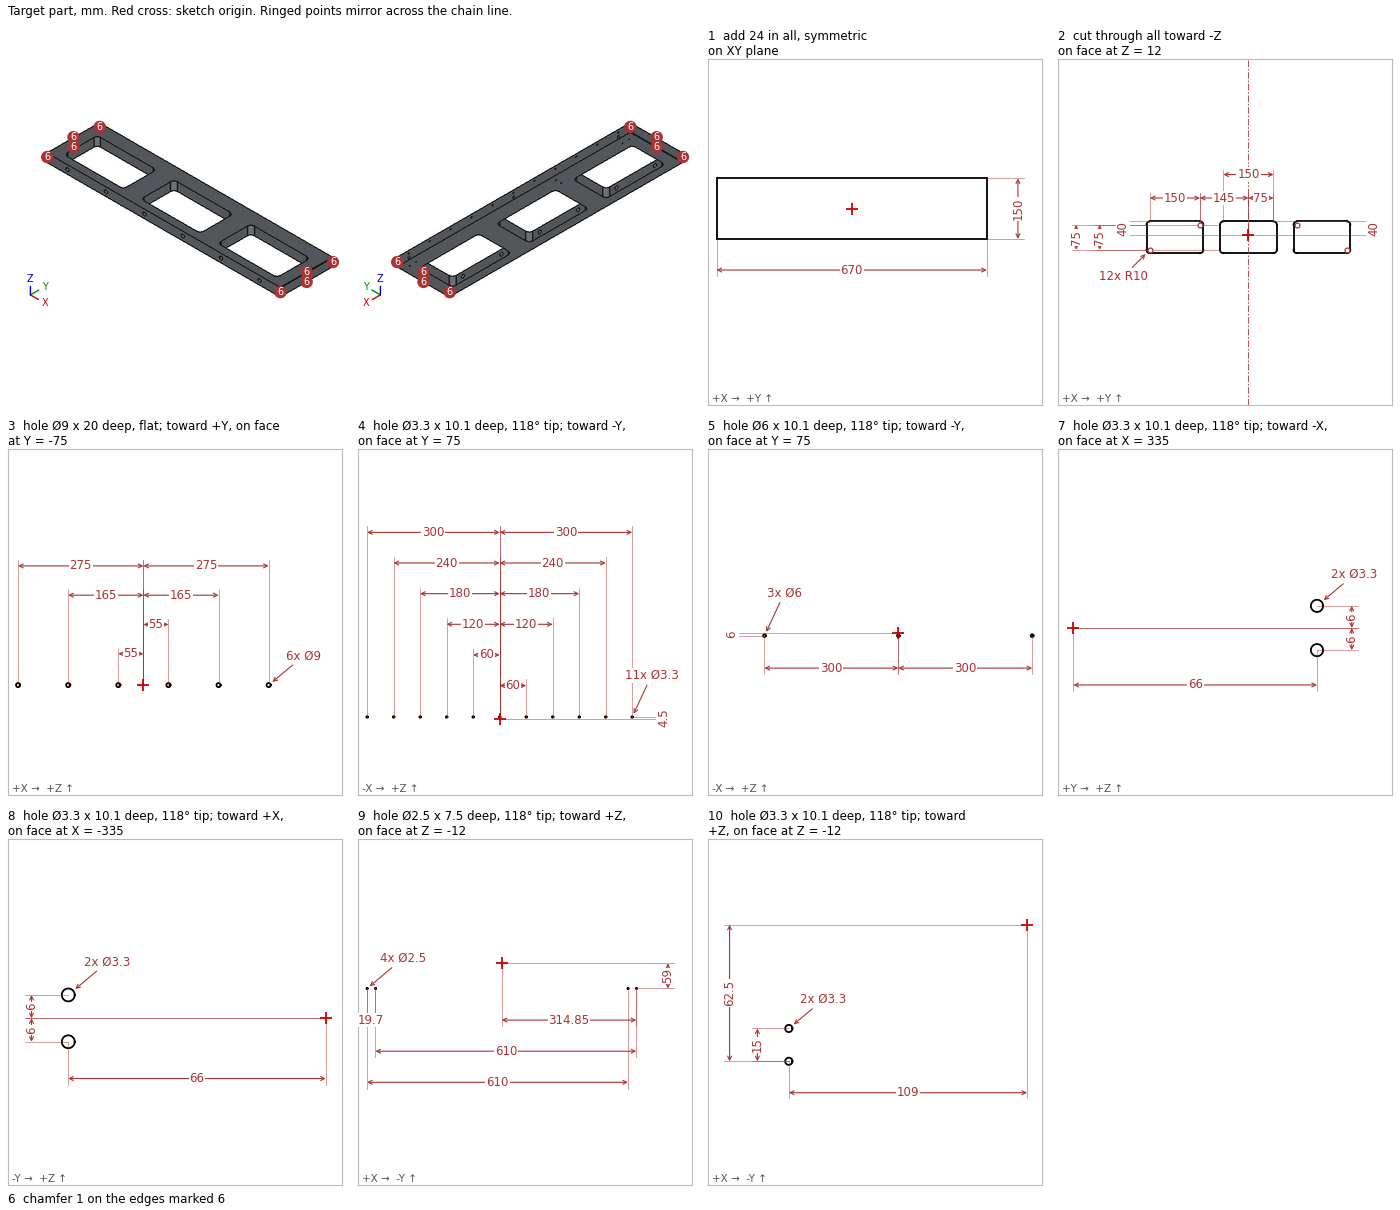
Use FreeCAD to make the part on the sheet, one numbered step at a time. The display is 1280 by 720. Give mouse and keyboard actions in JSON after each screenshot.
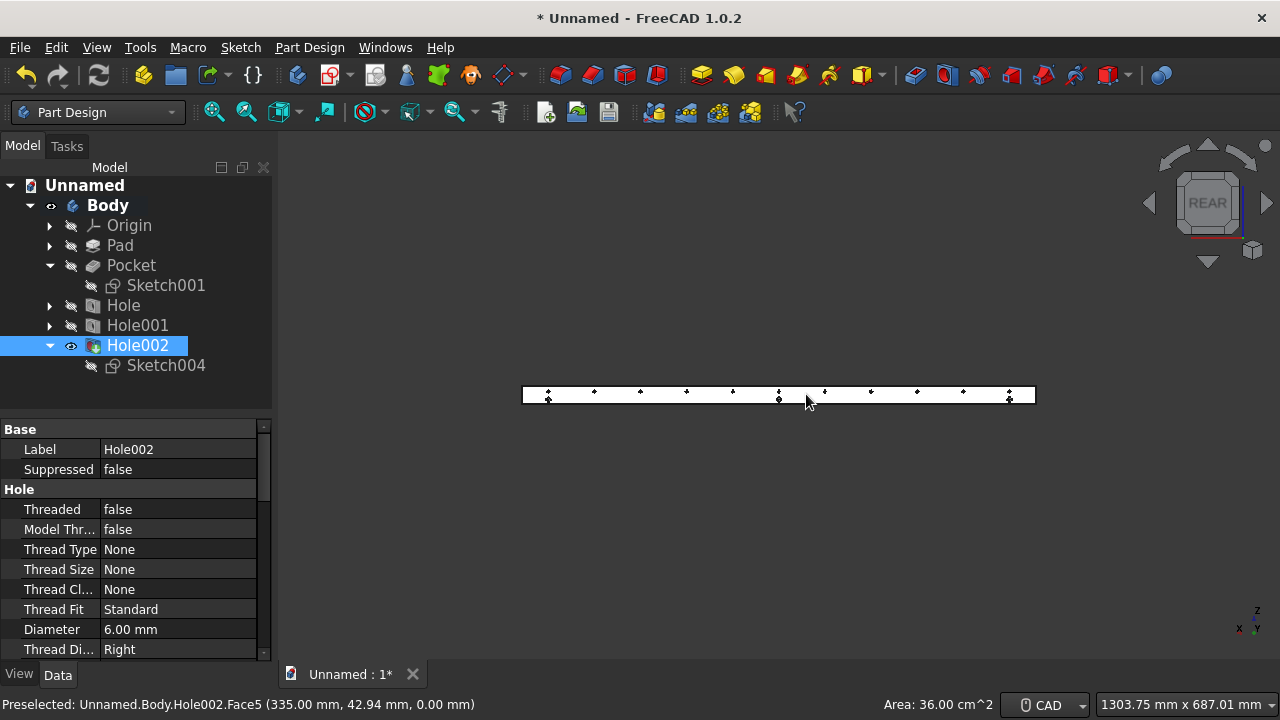
{"action": "key", "text": "6"}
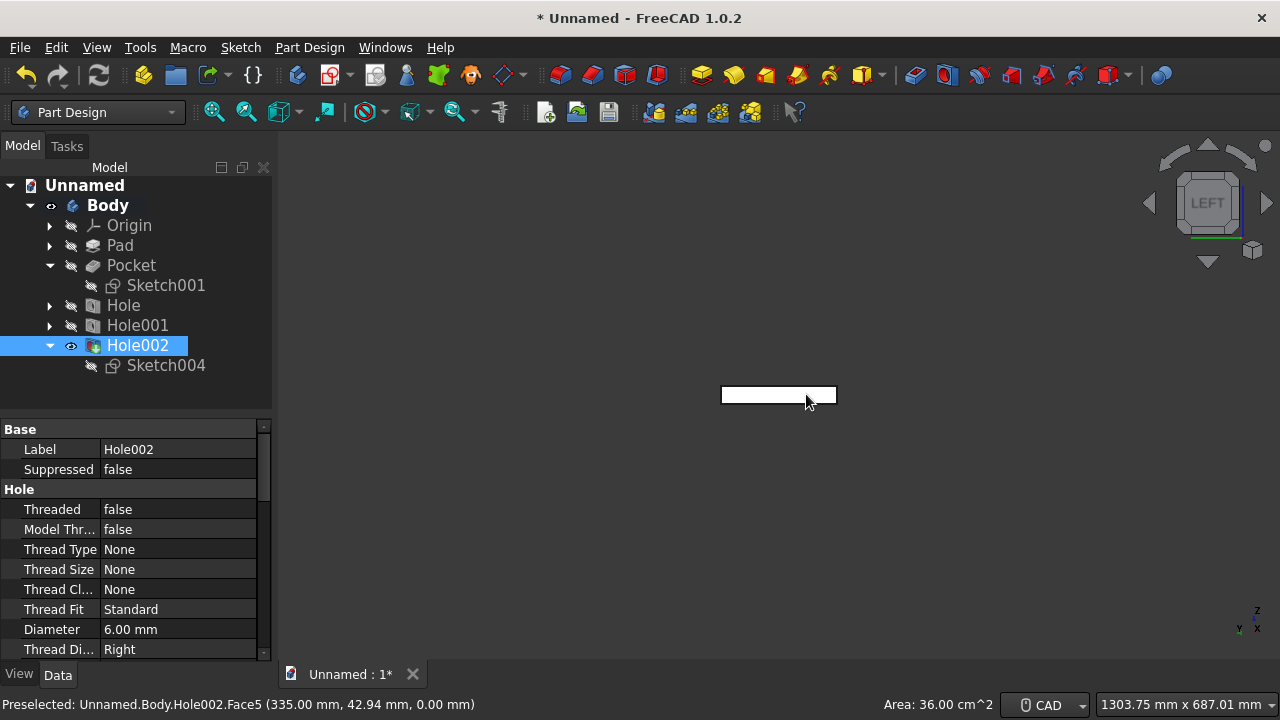
{"action": "left_click", "coordinate": [216, 112]}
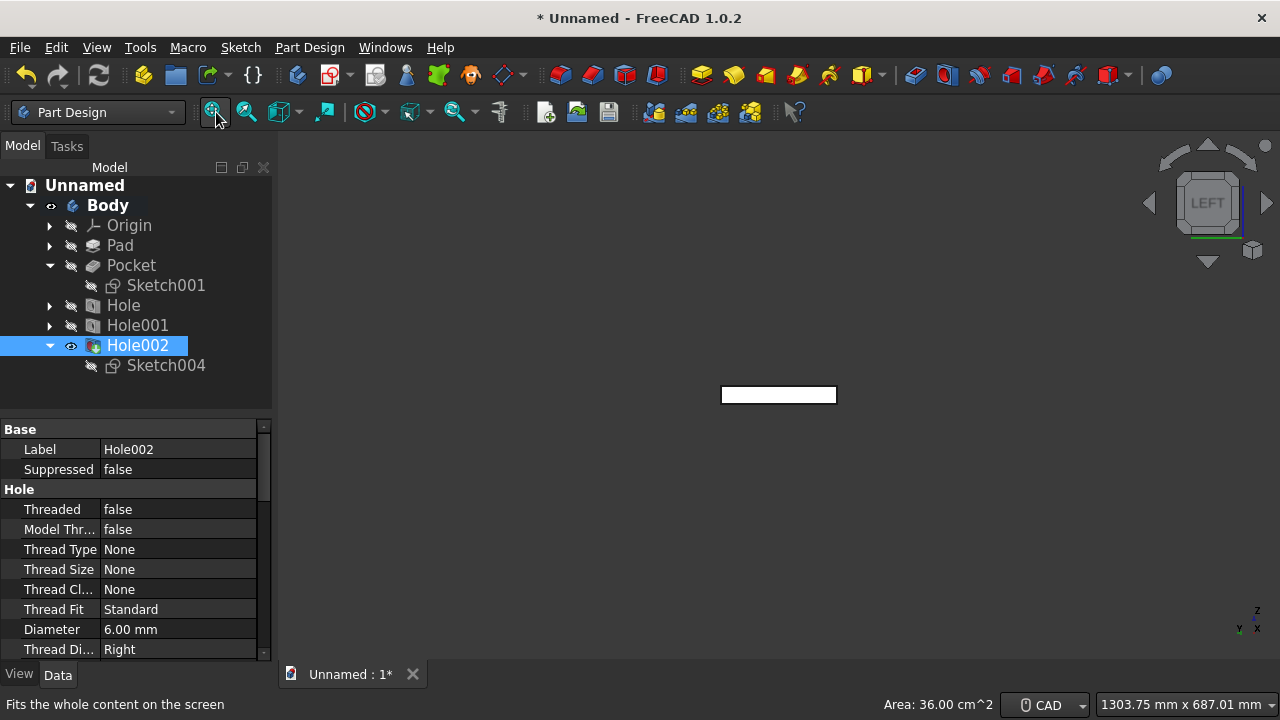
{"action": "left_click", "coordinate": [746, 394], "text": "ctrl"}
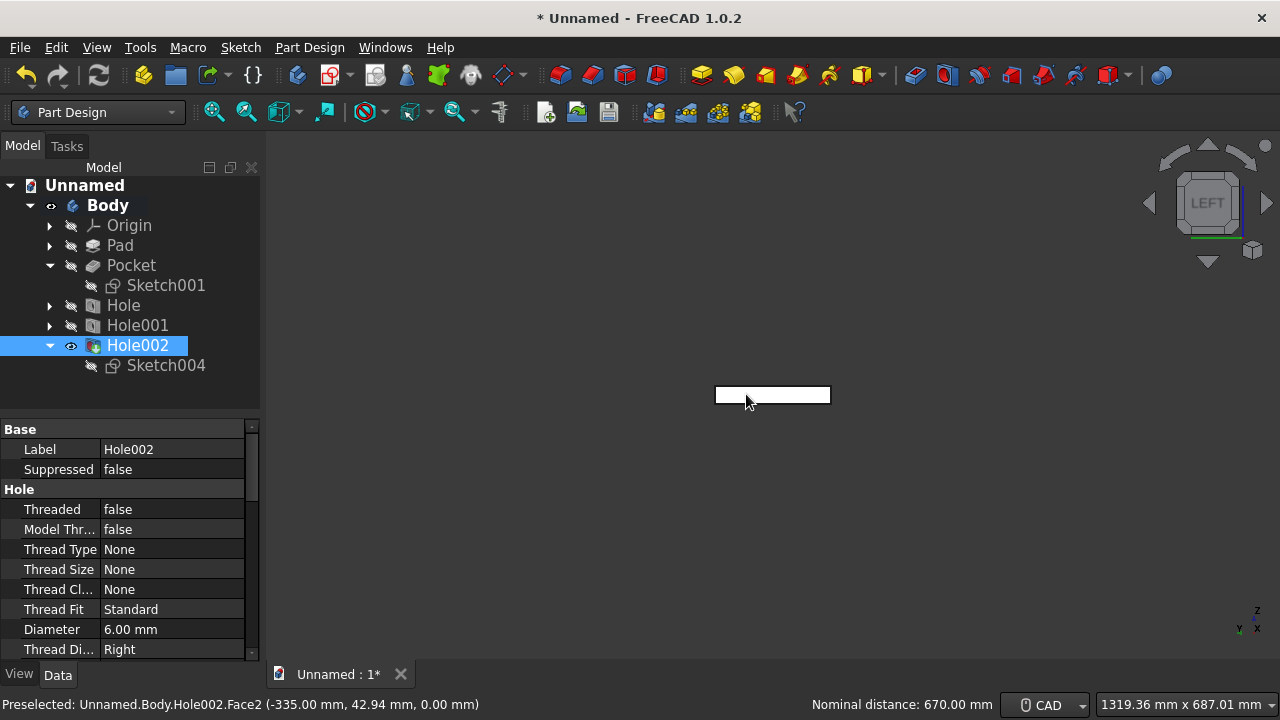
{"action": "left_click", "coordinate": [594, 76]}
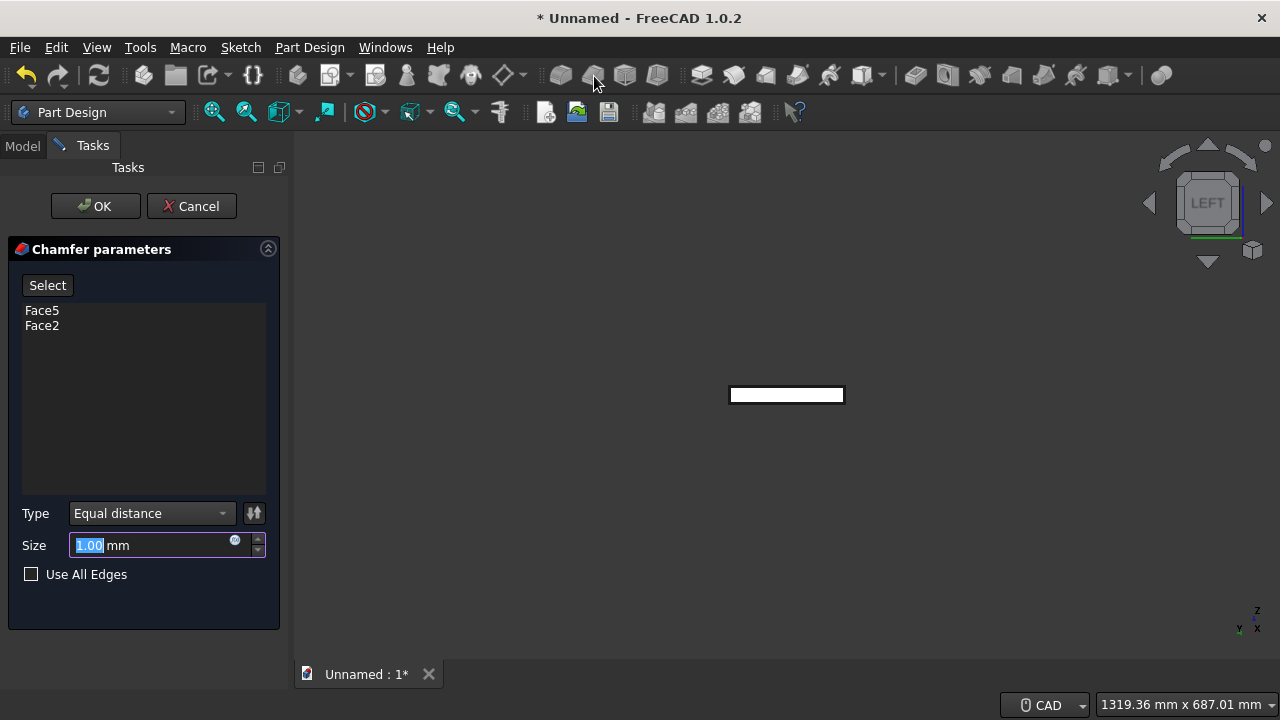
{"action": "type", "text": "1"}
{"action": "key", "text": "Tab"}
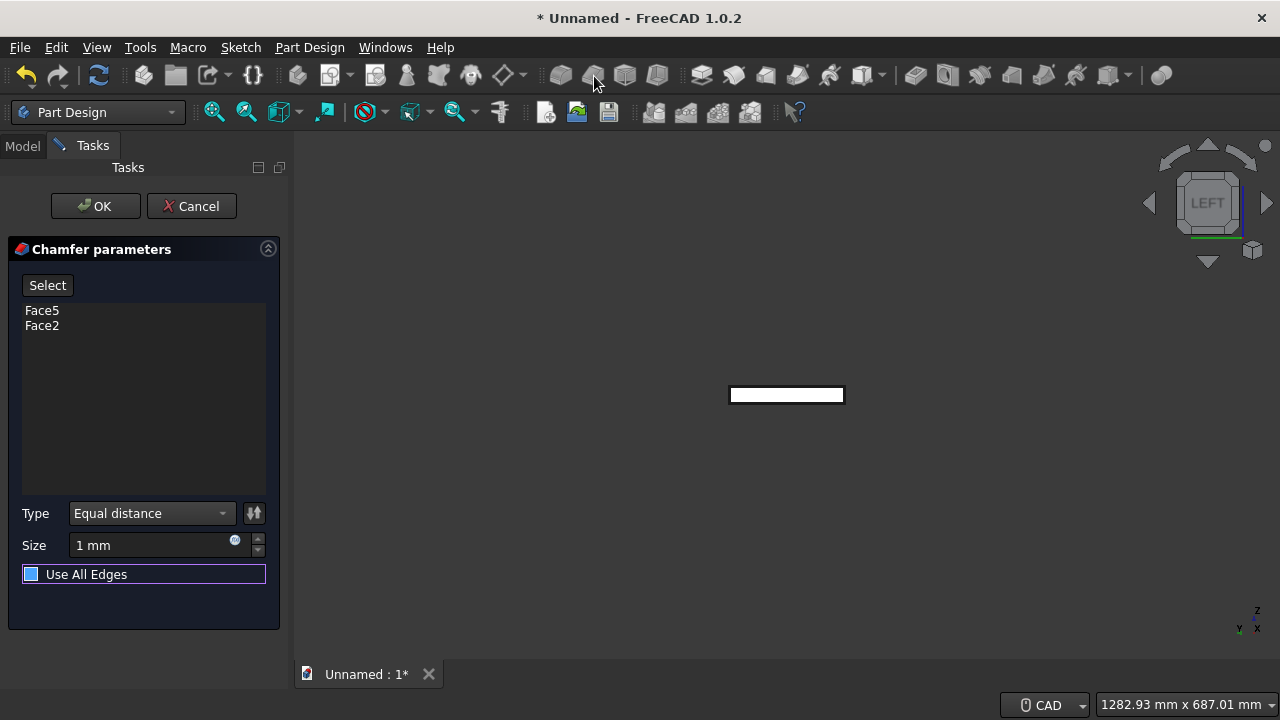
{"action": "left_click", "coordinate": [96, 206]}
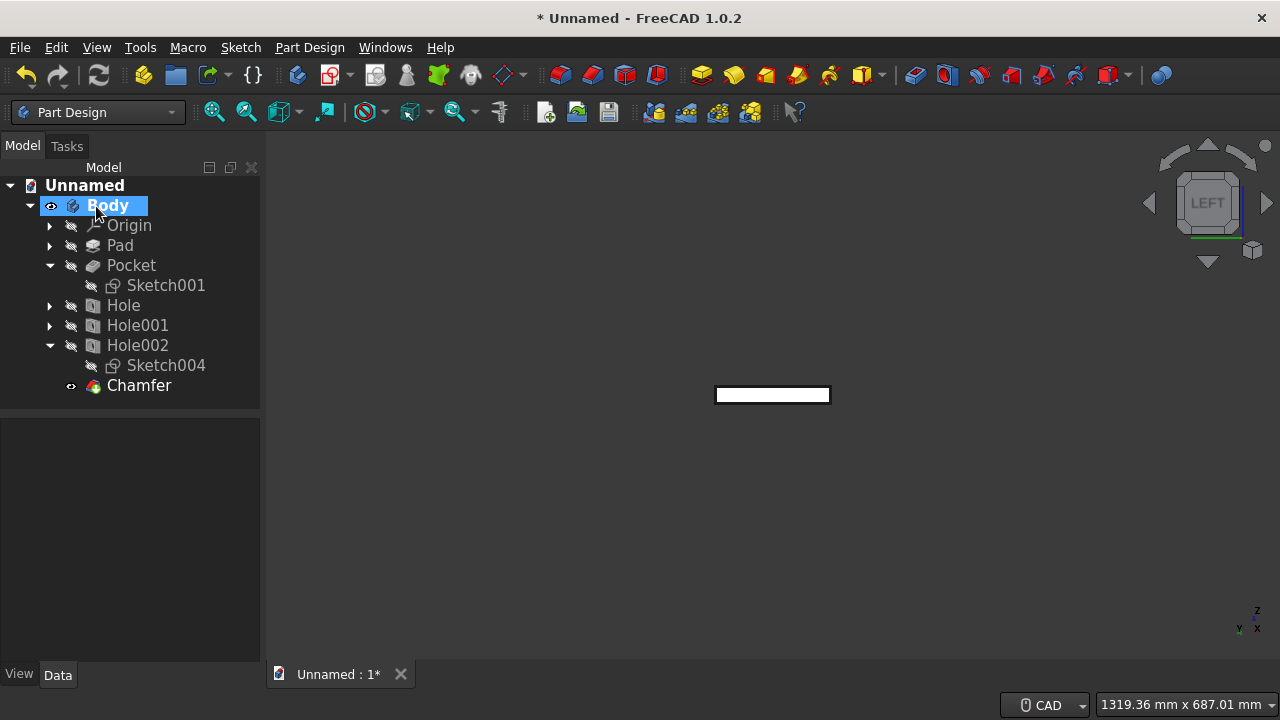
{"action": "left_click", "coordinate": [216, 112]}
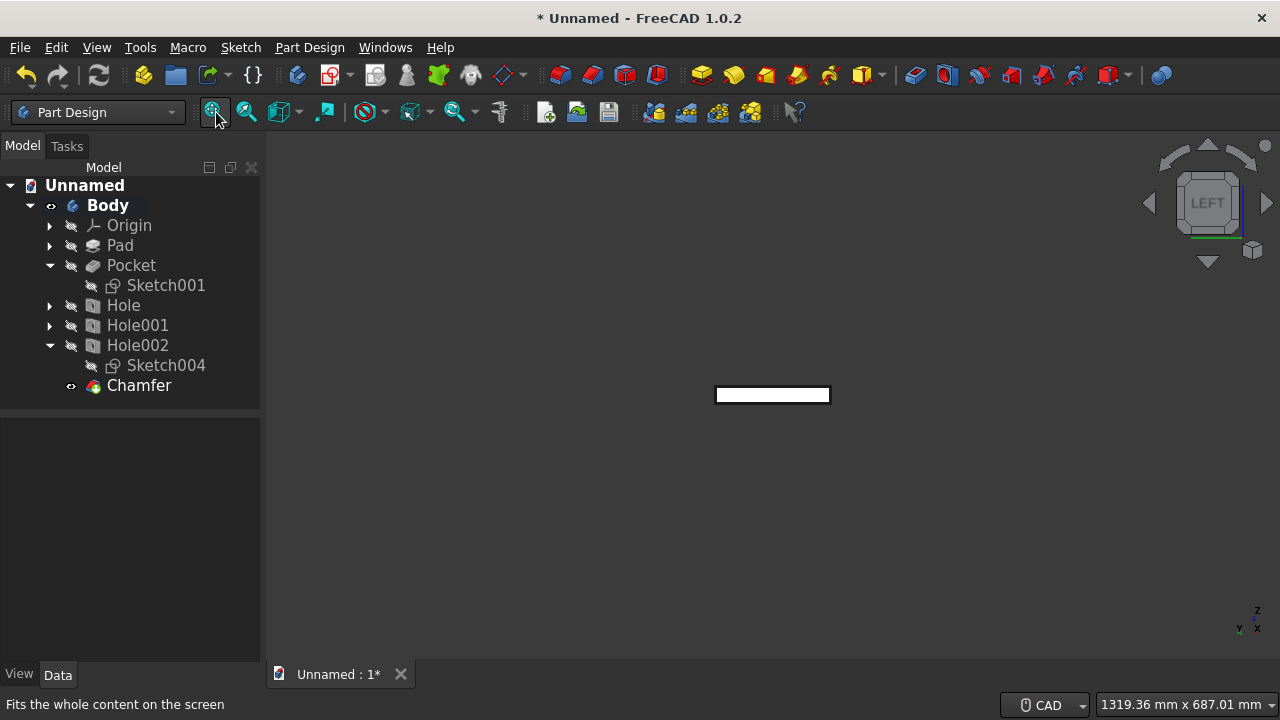
{"action": "key", "text": "0"}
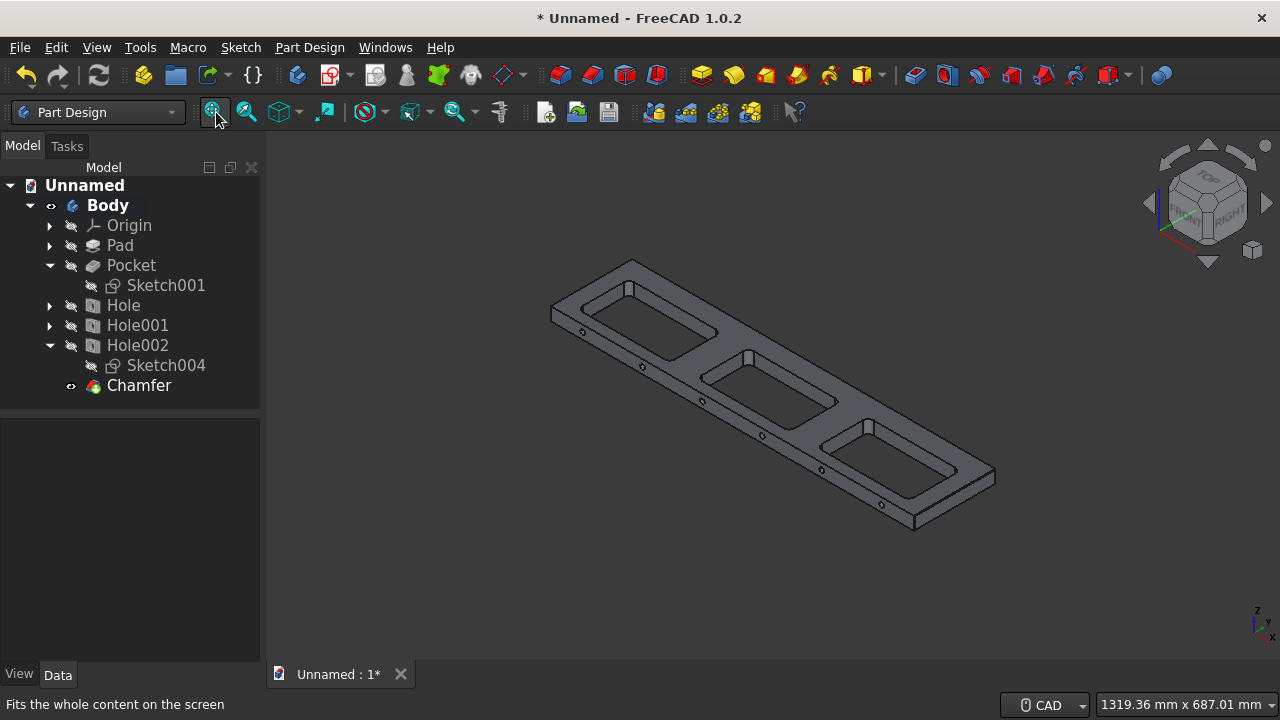
{"action": "key", "text": "3"}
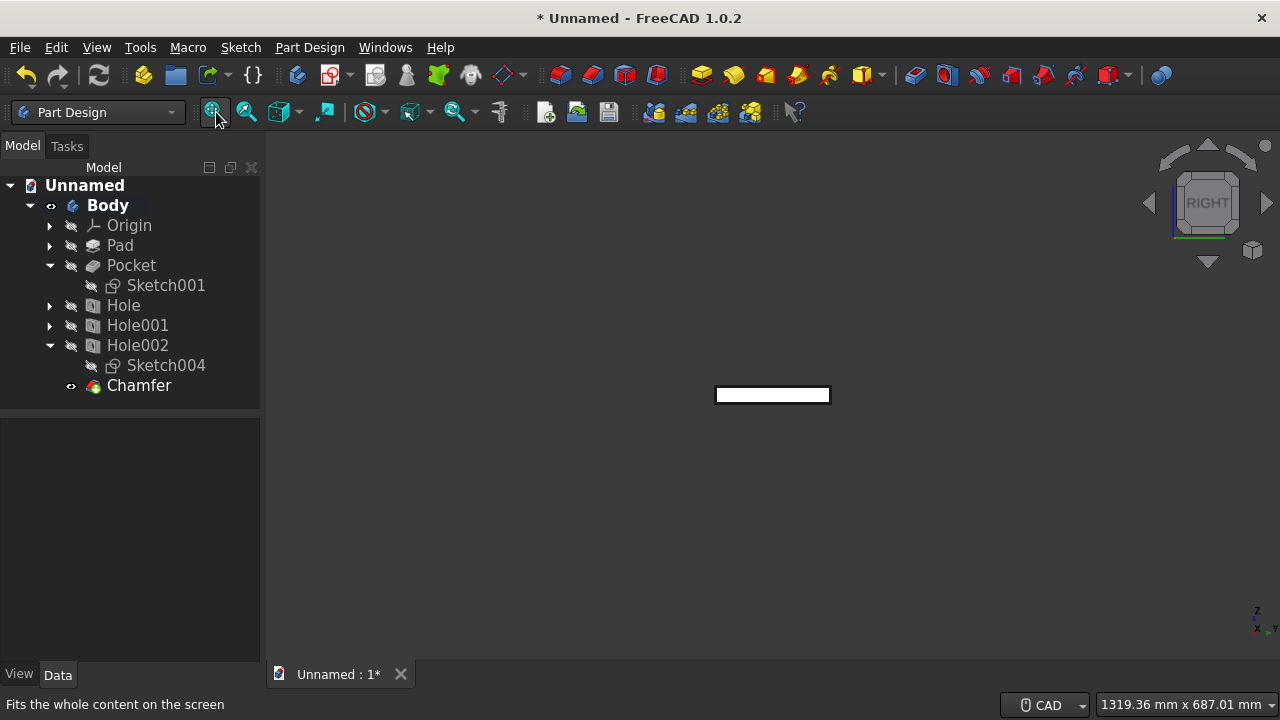
{"action": "left_click", "coordinate": [216, 112]}